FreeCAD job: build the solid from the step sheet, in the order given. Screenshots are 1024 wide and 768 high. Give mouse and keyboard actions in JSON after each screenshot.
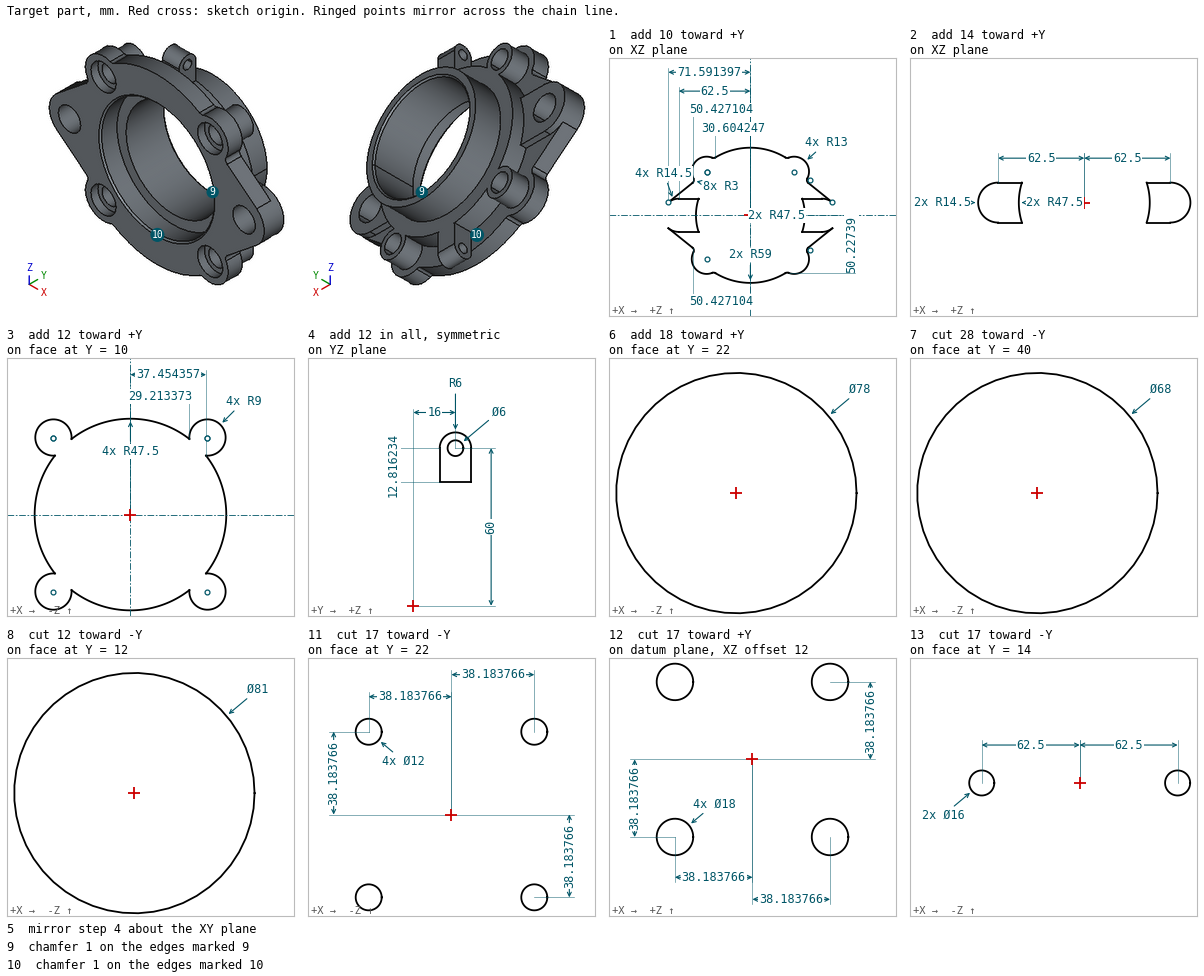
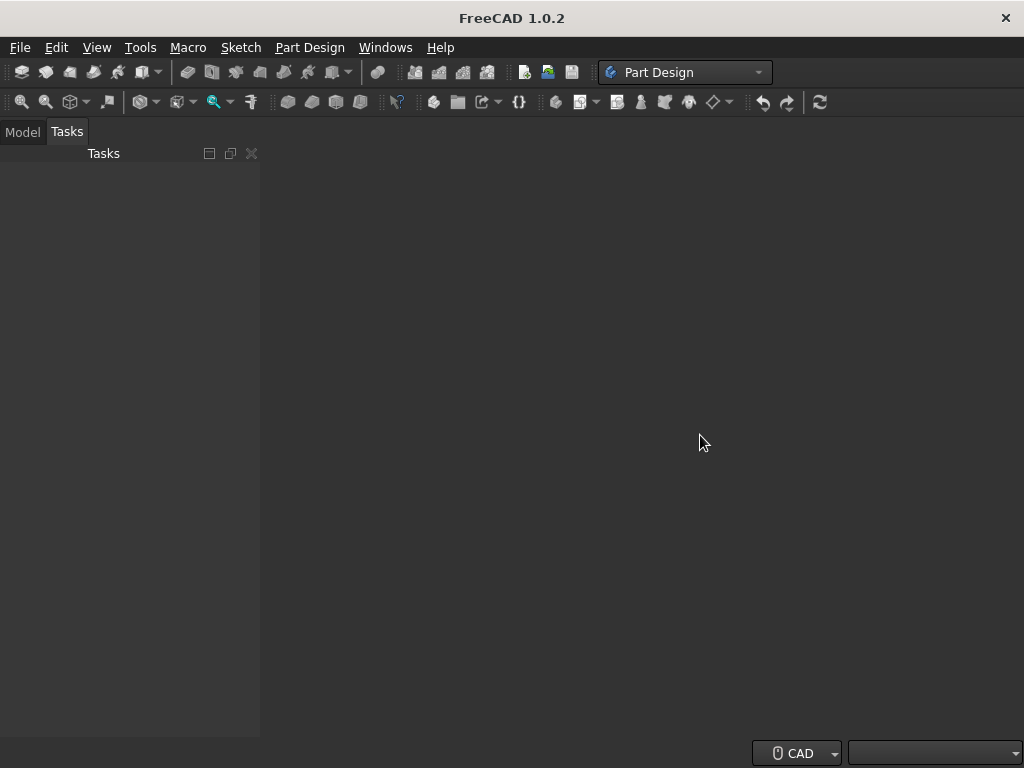
{"action": "key", "text": "ctrl+n"}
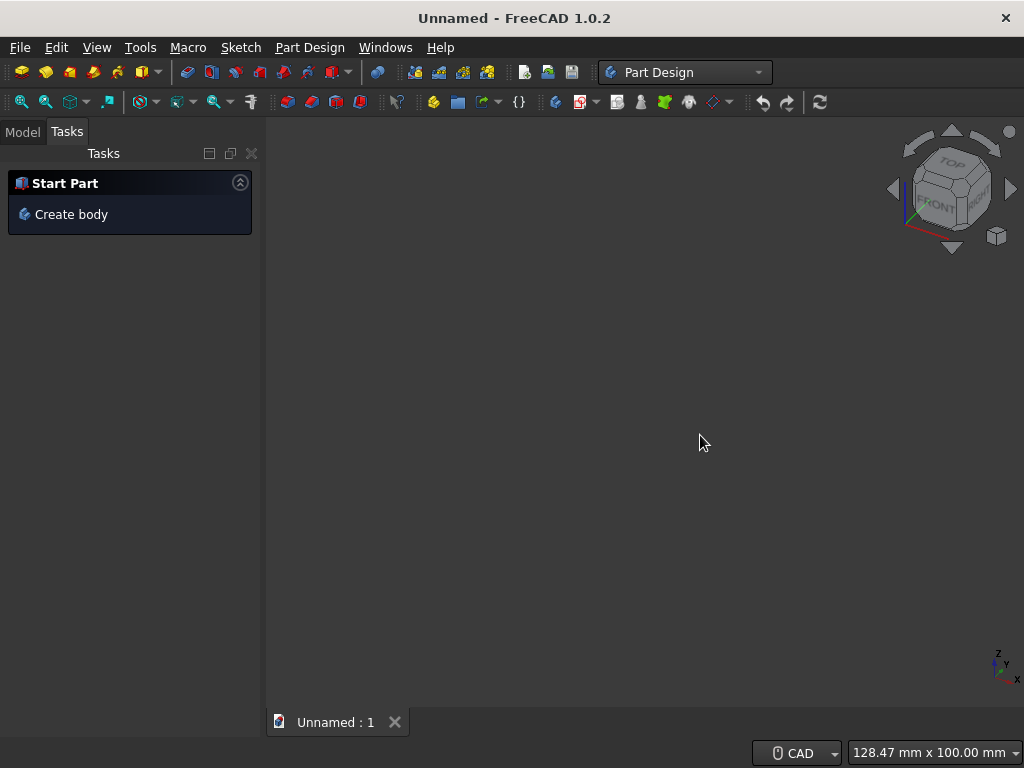
{"action": "left_click", "coordinate": [580, 102]}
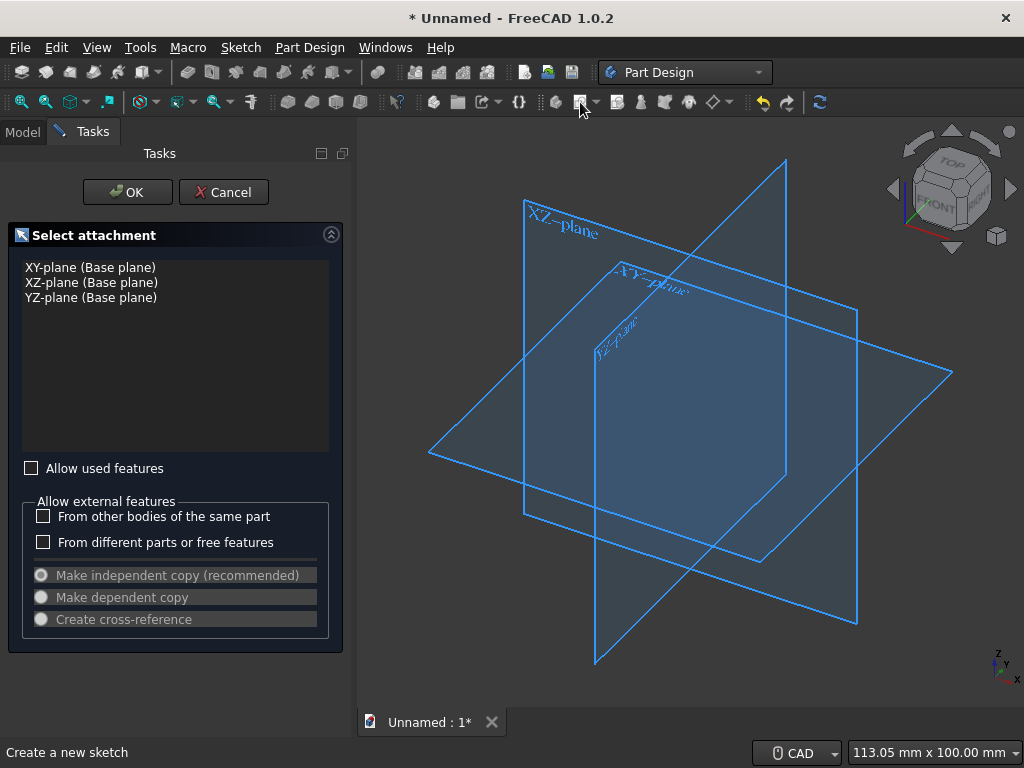
{"action": "left_click", "coordinate": [82, 282]}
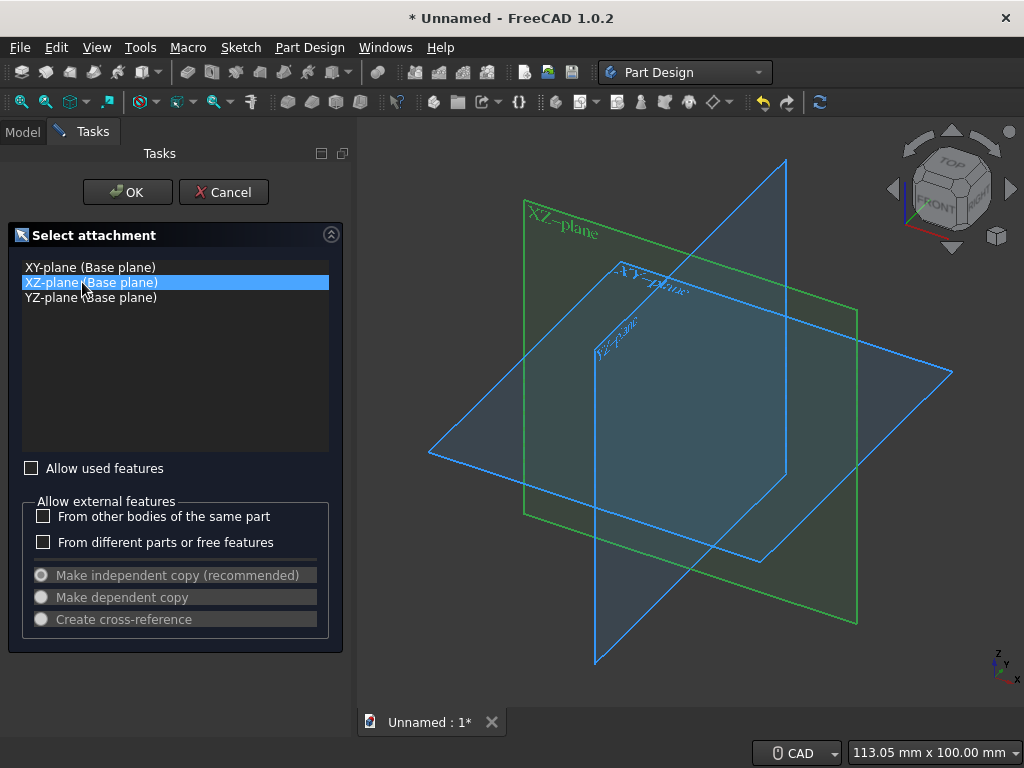
{"action": "left_click", "coordinate": [128, 192]}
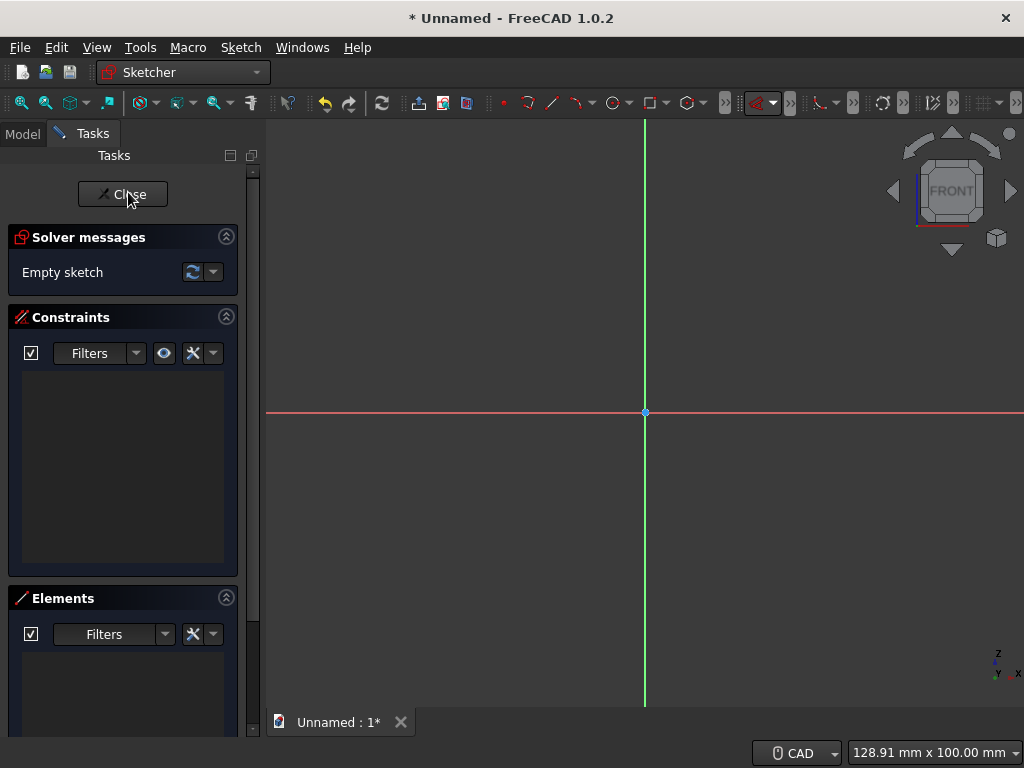
{"action": "scroll", "coordinate": [521, 413], "scroll_direction": "down", "scroll_amount": 4}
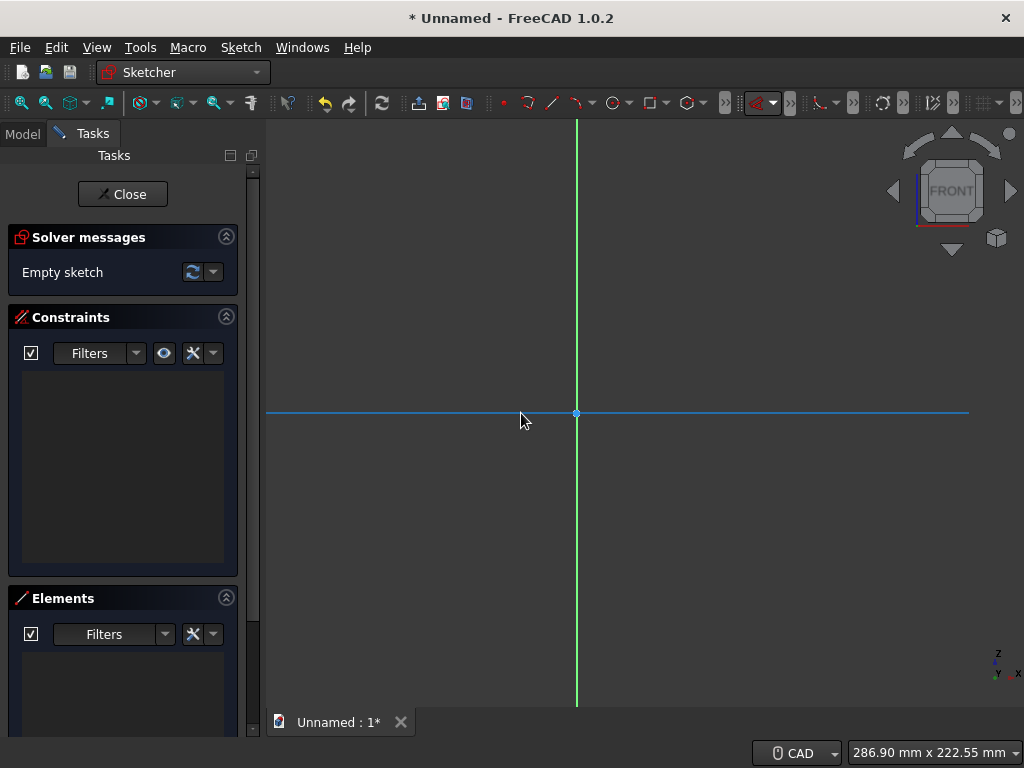
{"action": "left_click", "coordinate": [552, 104]}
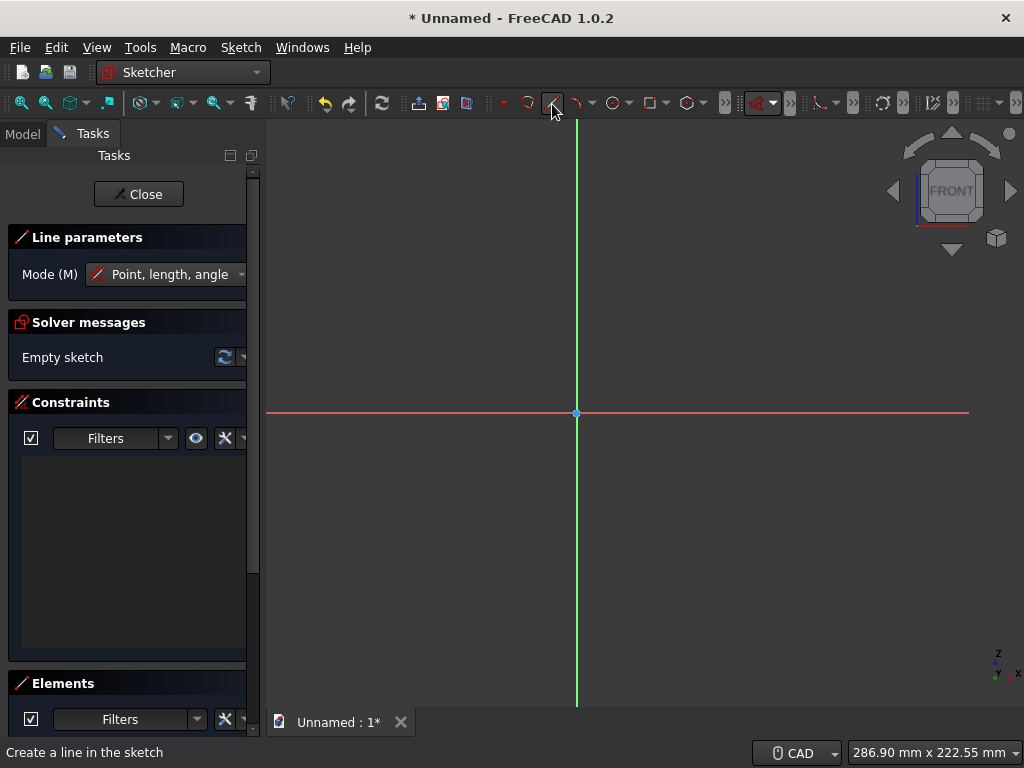
{"action": "left_click", "coordinate": [457, 375]}
{"action": "left_click", "coordinate": [412, 375]}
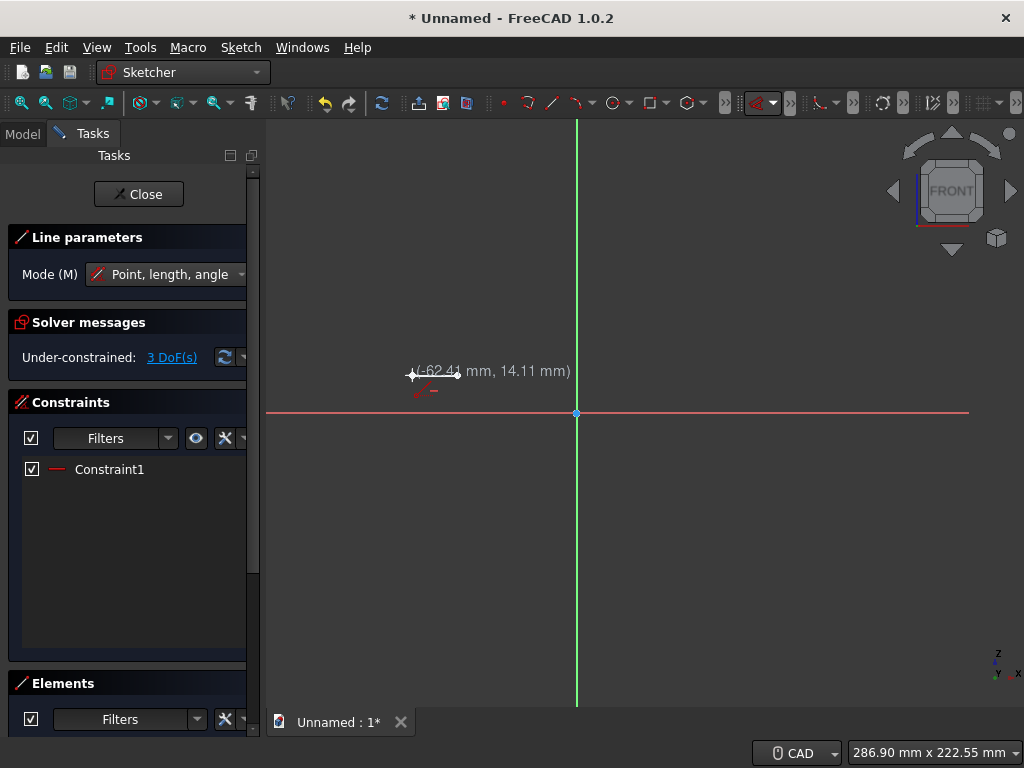
{"action": "left_click", "coordinate": [388, 383]}
{"action": "left_click", "coordinate": [444, 338]}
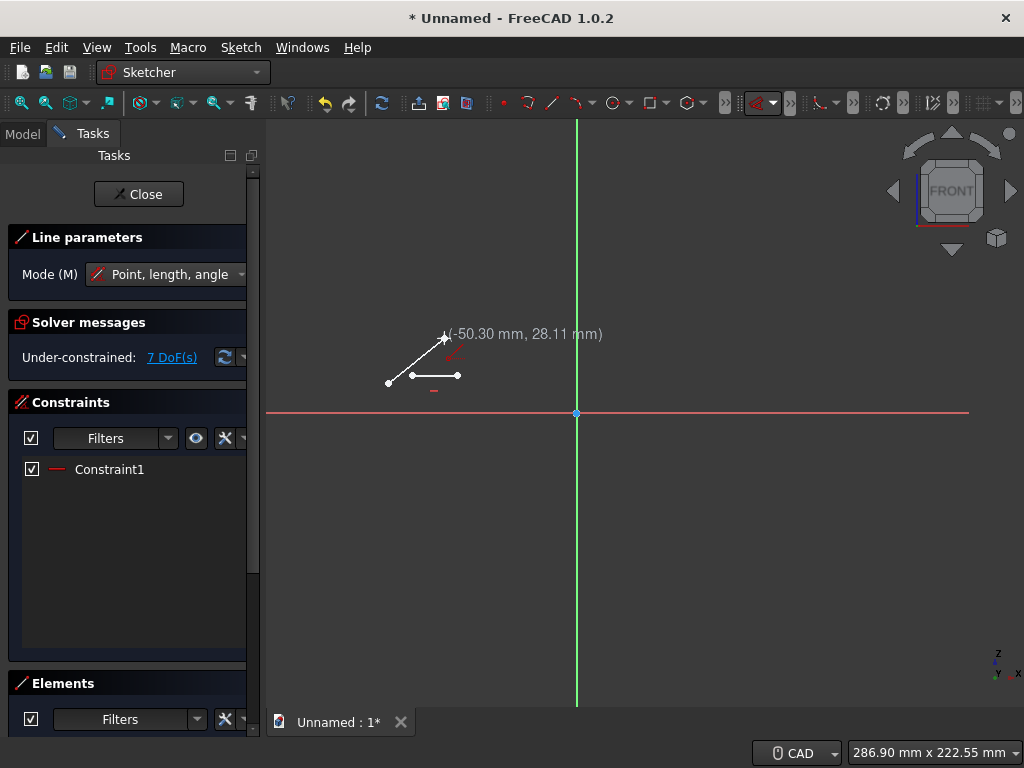
{"action": "left_click", "coordinate": [710, 338]}
{"action": "left_click", "coordinate": [766, 383]}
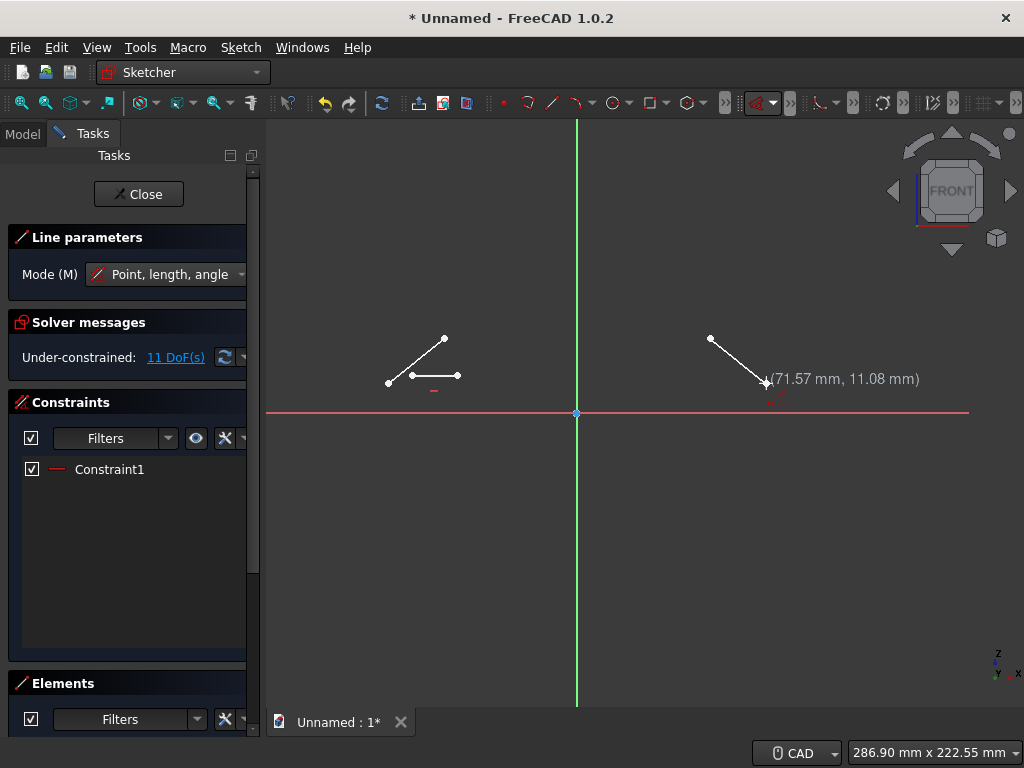
{"action": "scroll", "coordinate": [742, 375], "scroll_direction": "up", "scroll_amount": 4}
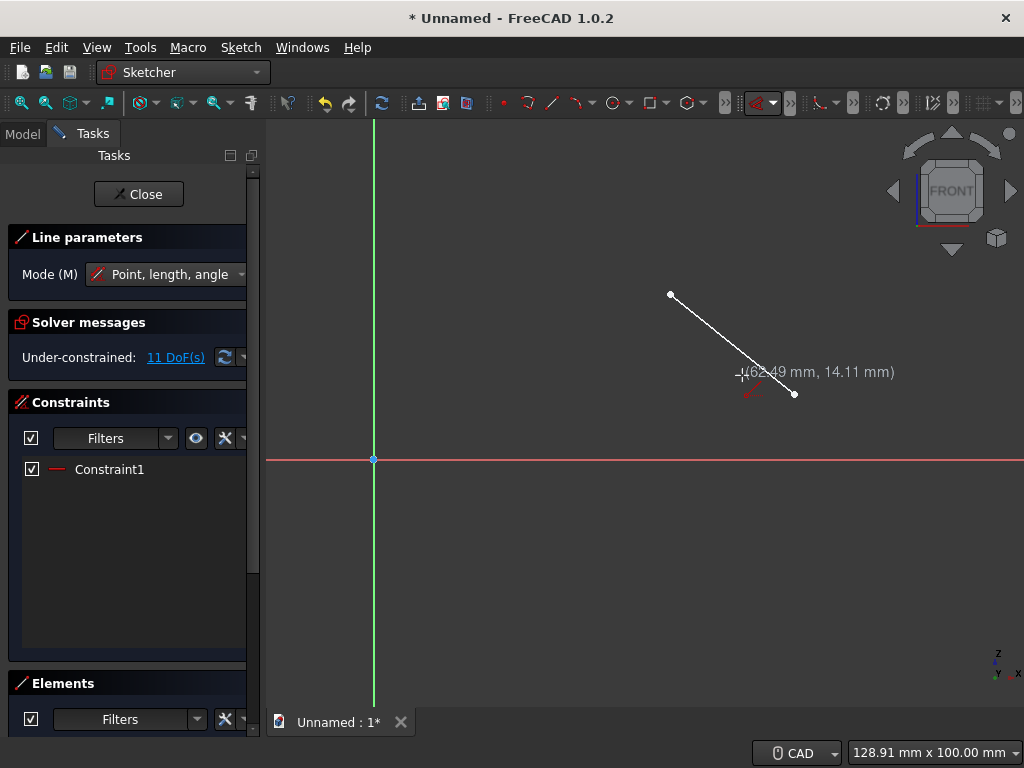
{"action": "left_click", "coordinate": [741, 374]}
{"action": "left_click", "coordinate": [640, 374]}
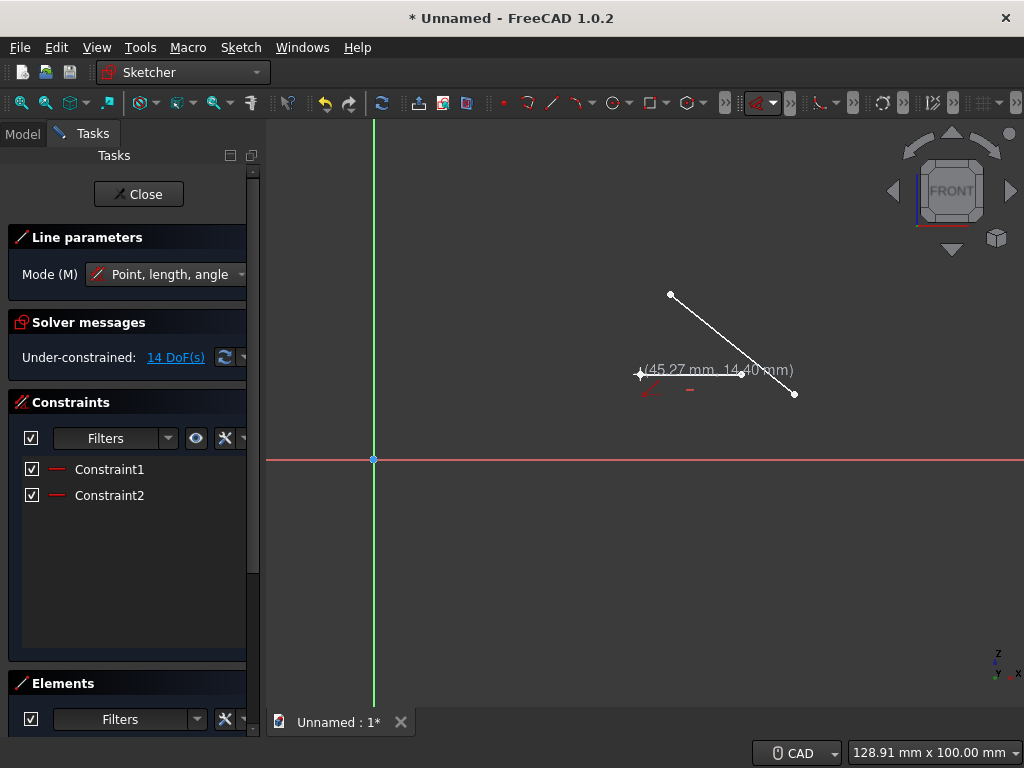
{"action": "left_click", "coordinate": [640, 545]}
{"action": "left_click", "coordinate": [741, 545]}